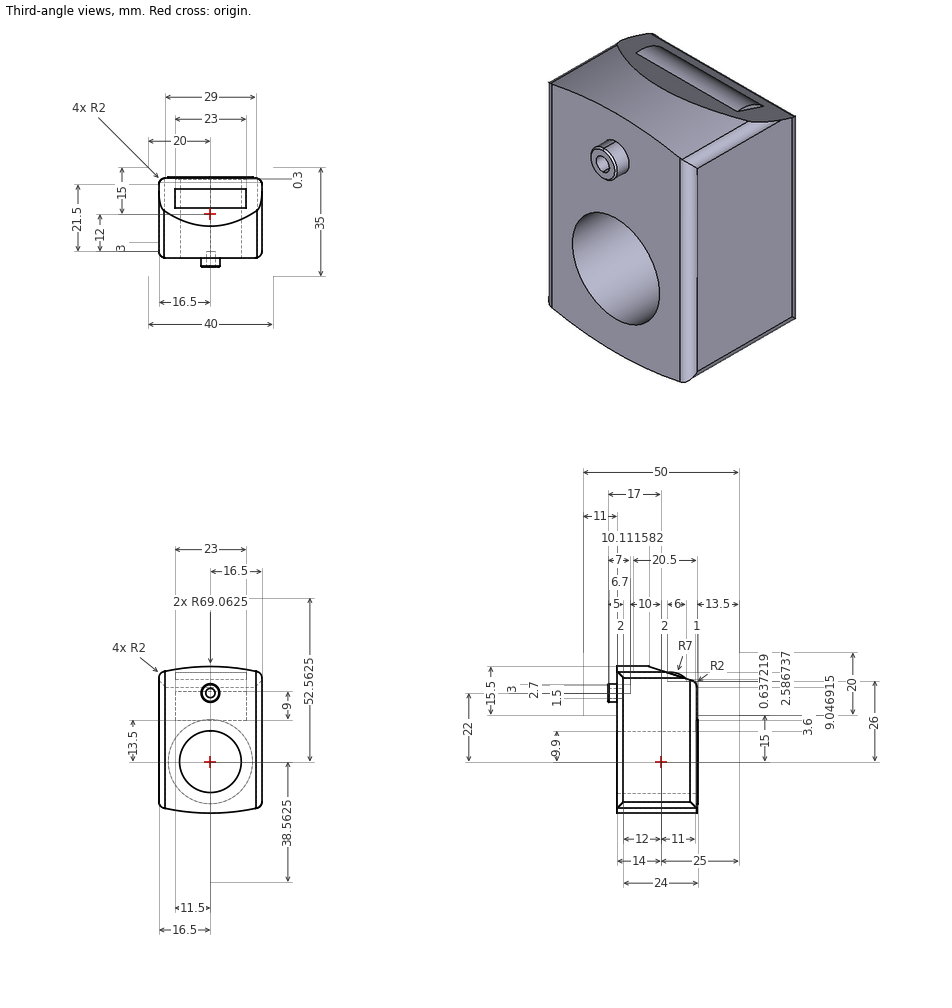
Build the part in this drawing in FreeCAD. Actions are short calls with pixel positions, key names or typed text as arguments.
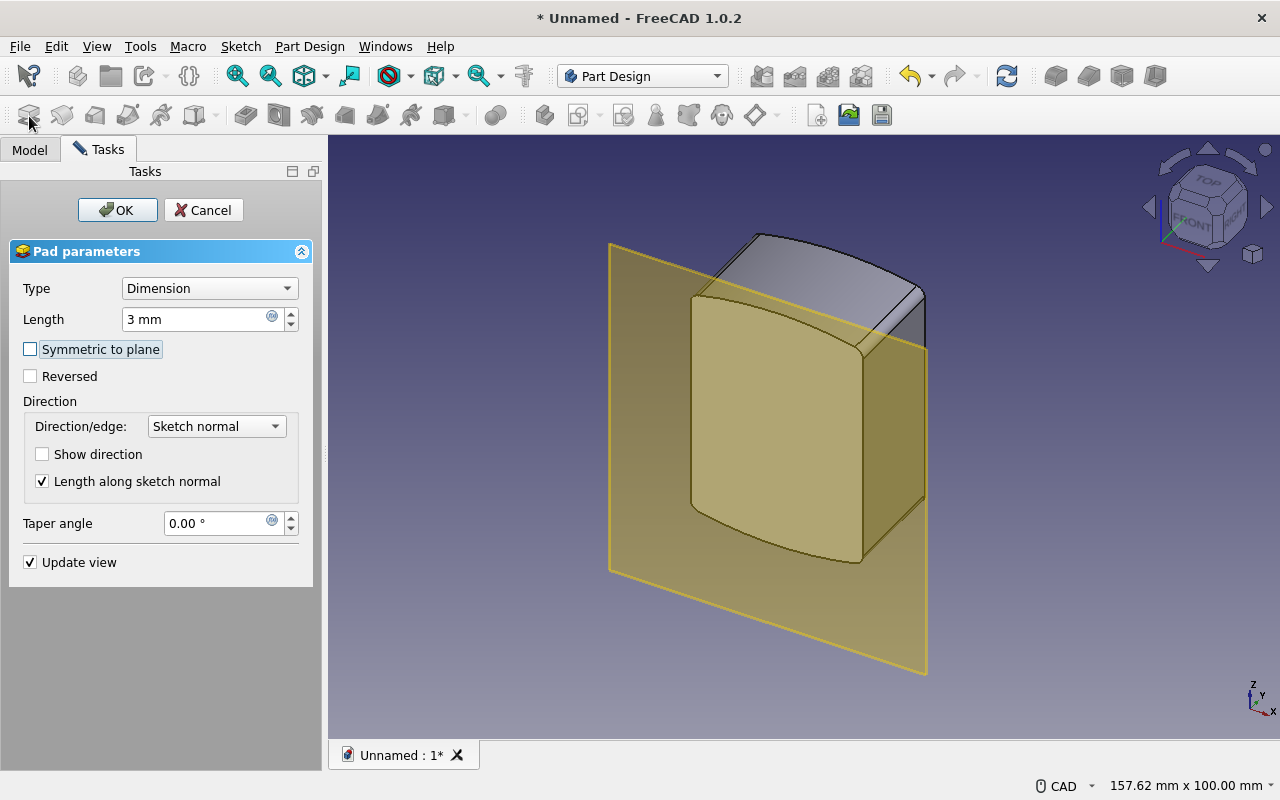
click(31, 376)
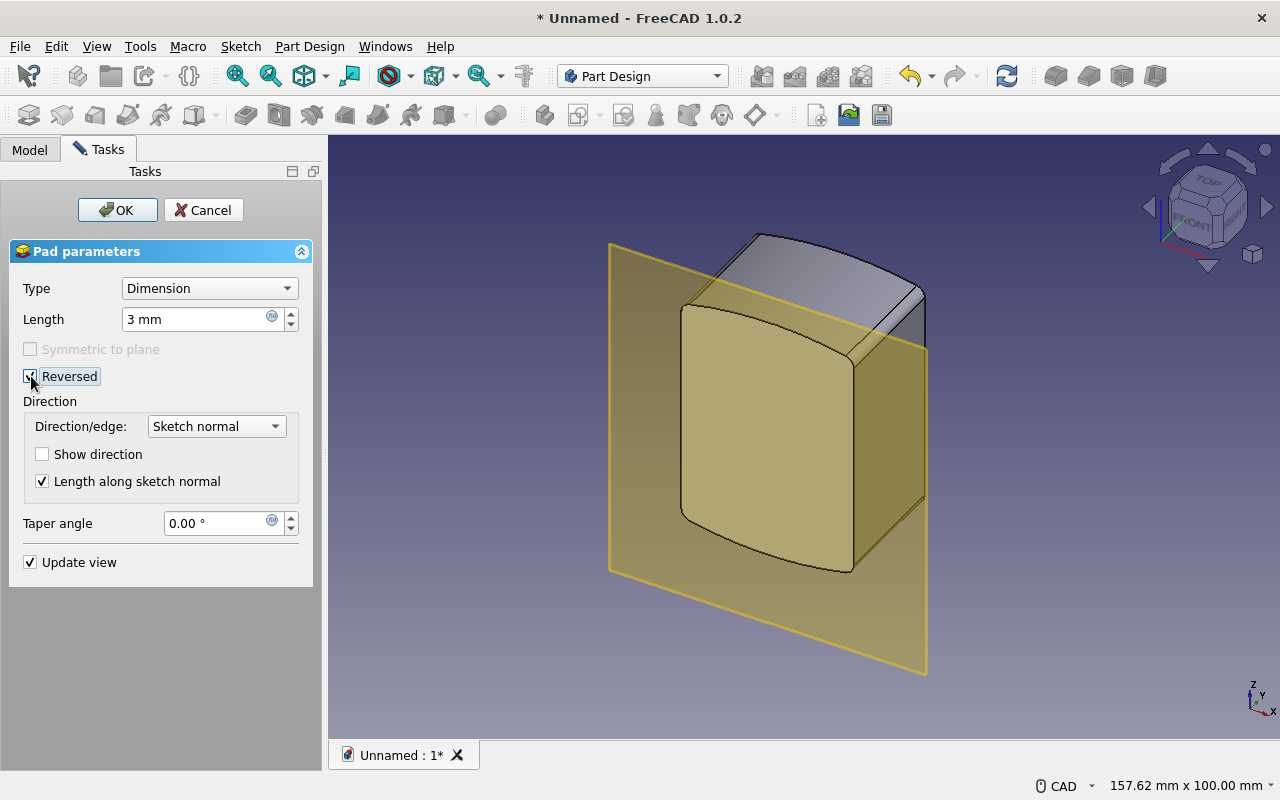
click(118, 210)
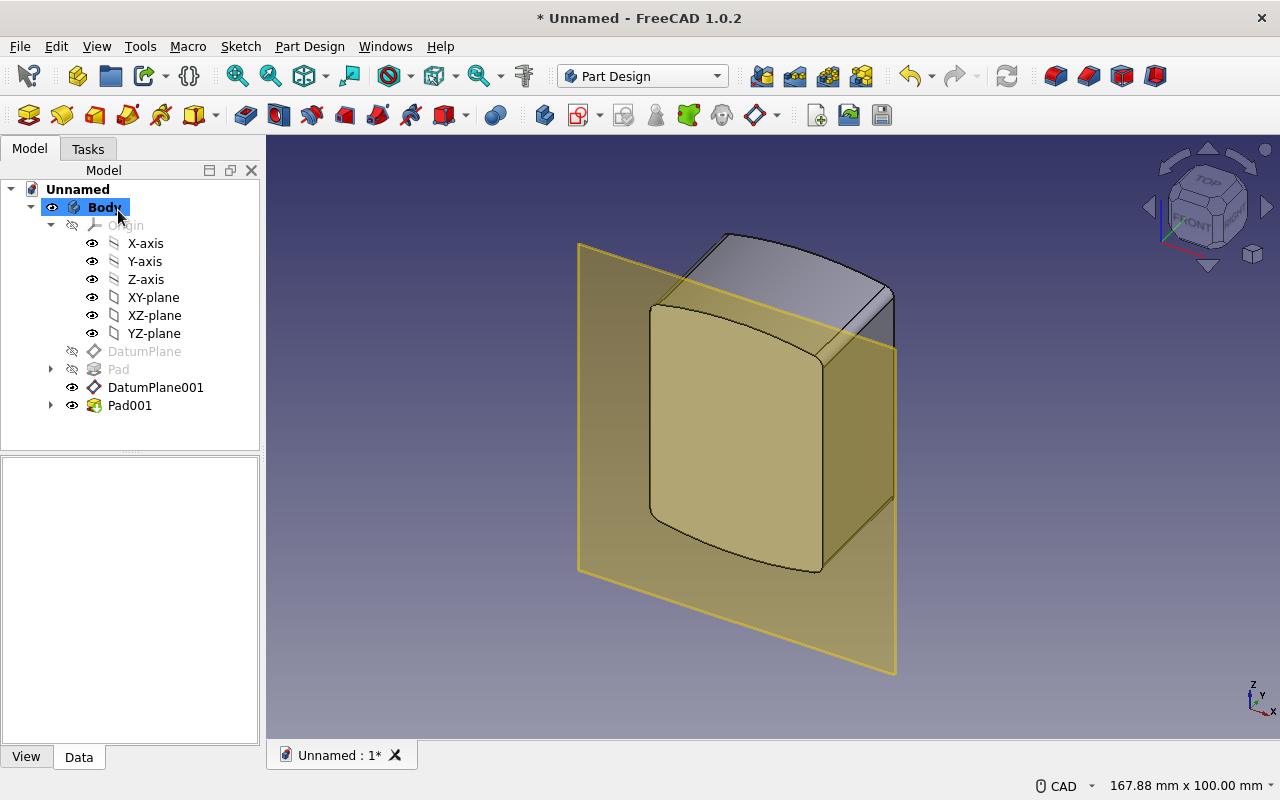
click(117, 387)
key(space)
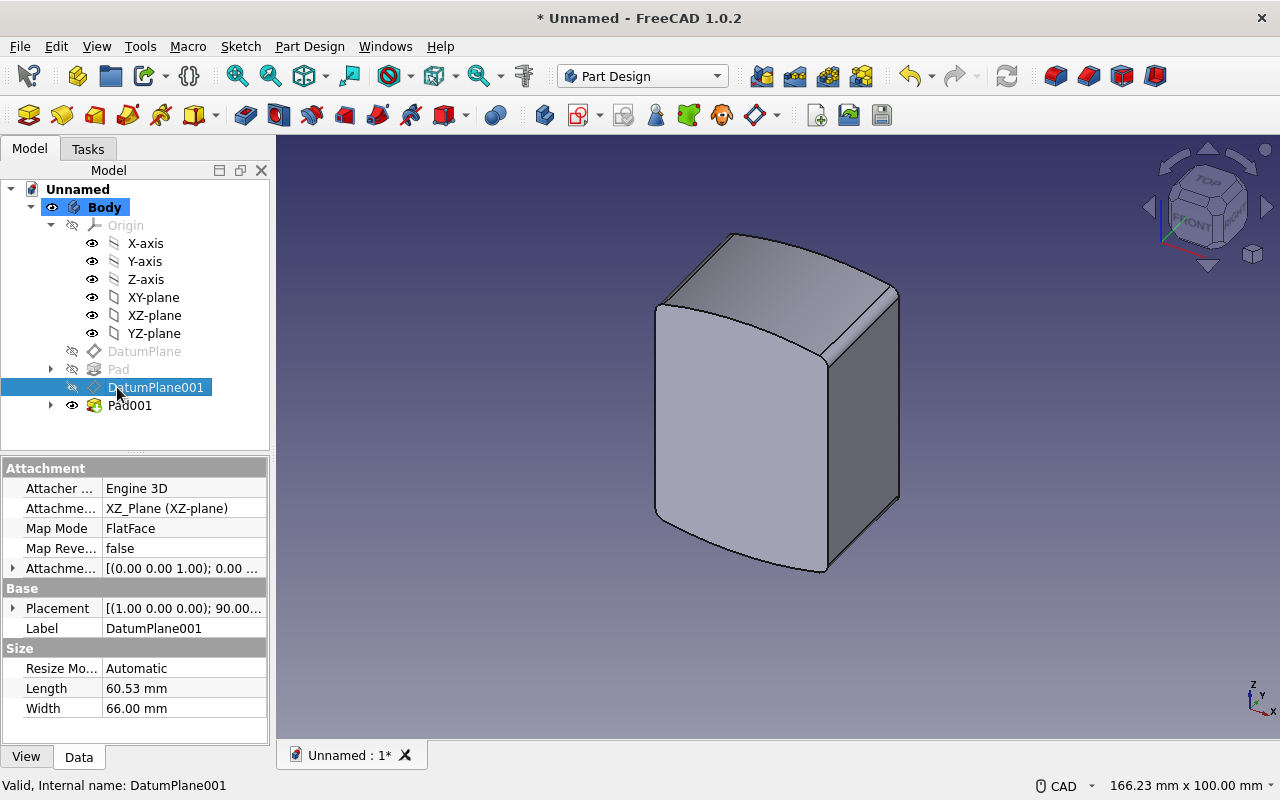
click(137, 315)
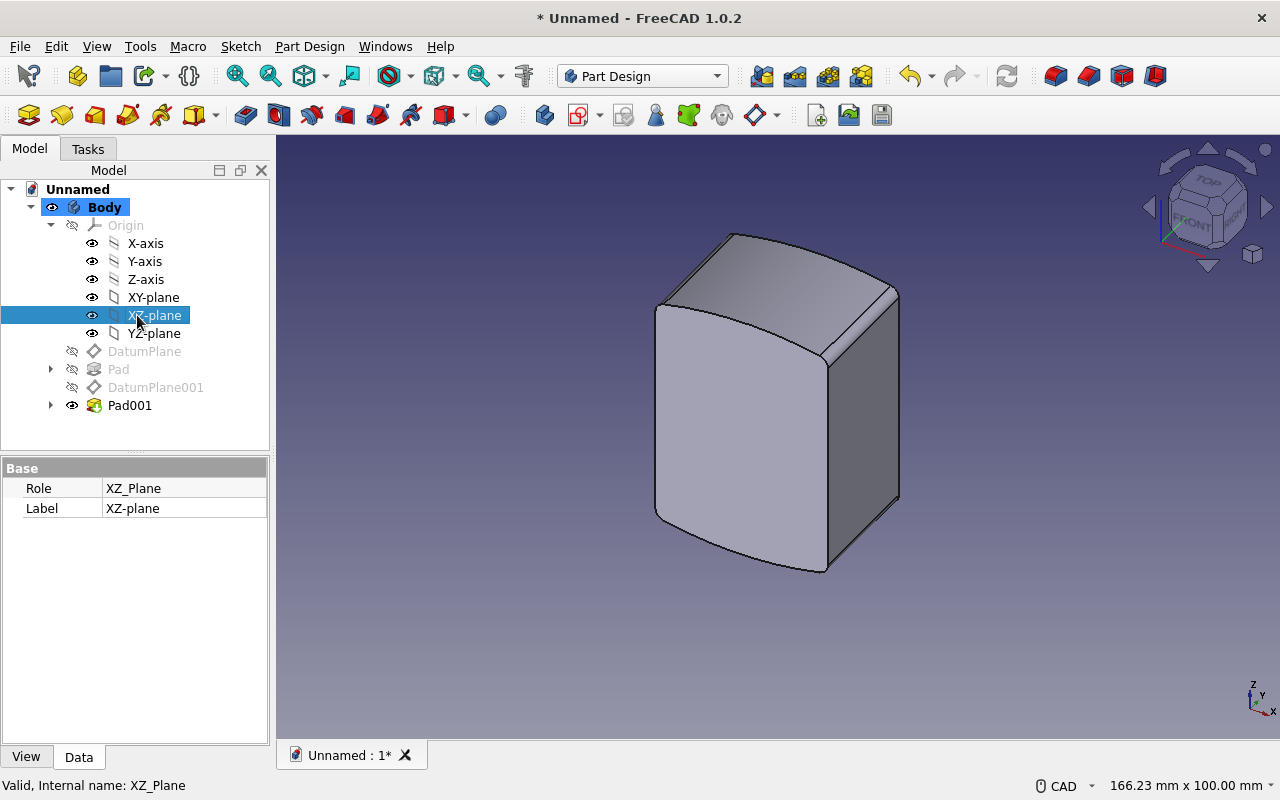
click(754, 116)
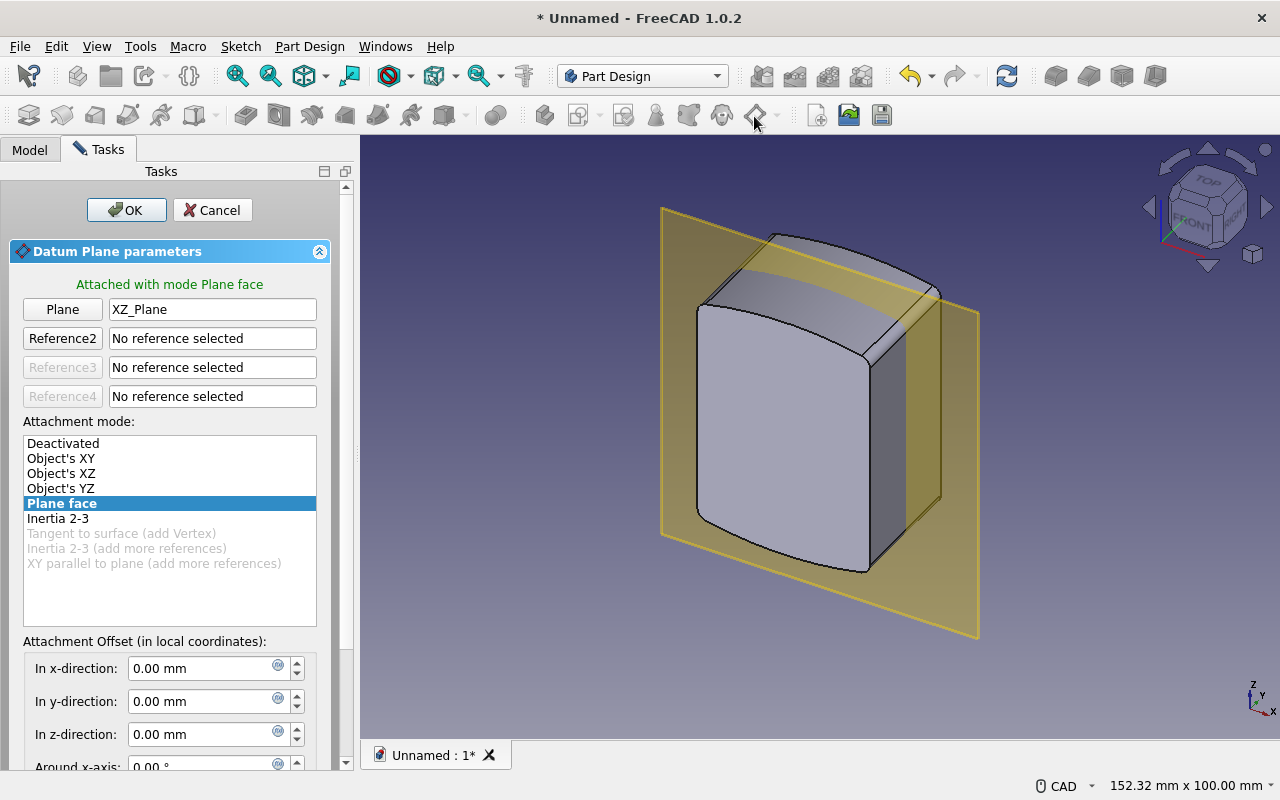
triple_click(210, 734)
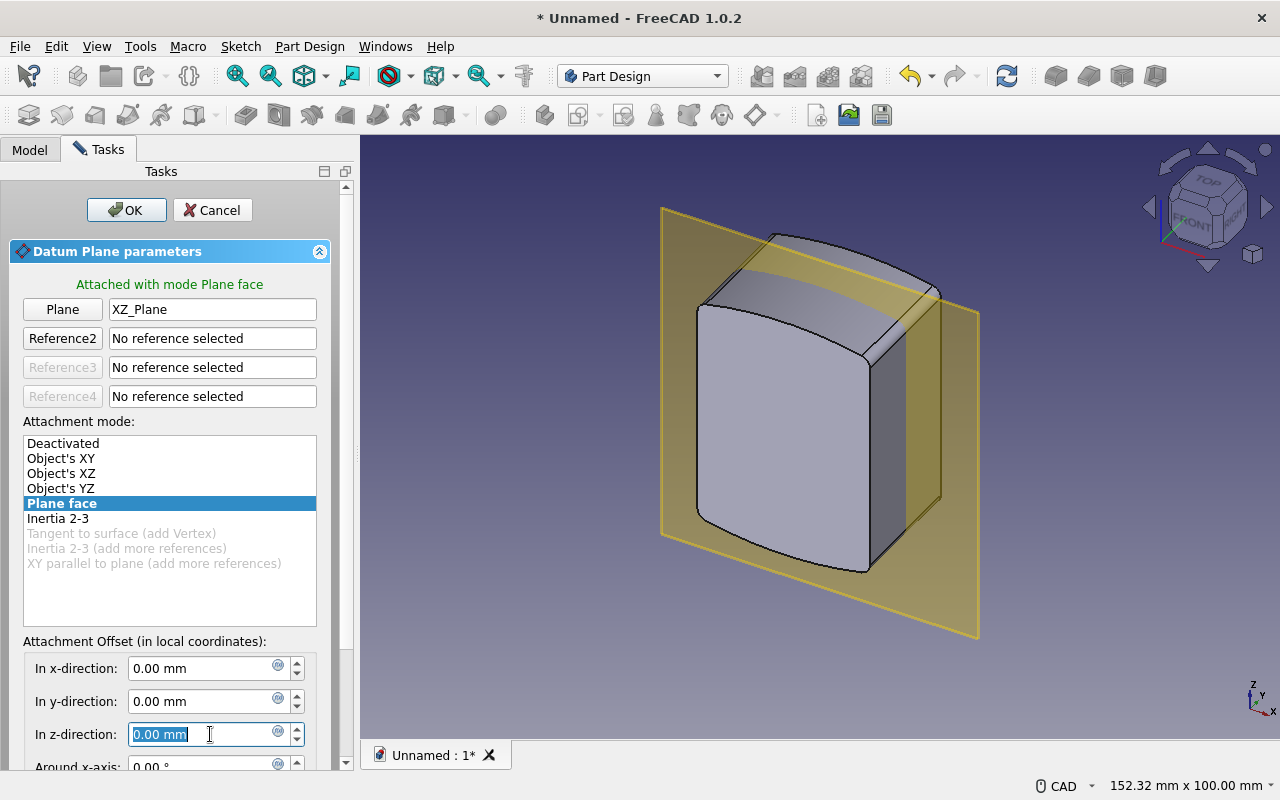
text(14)
key(Tab)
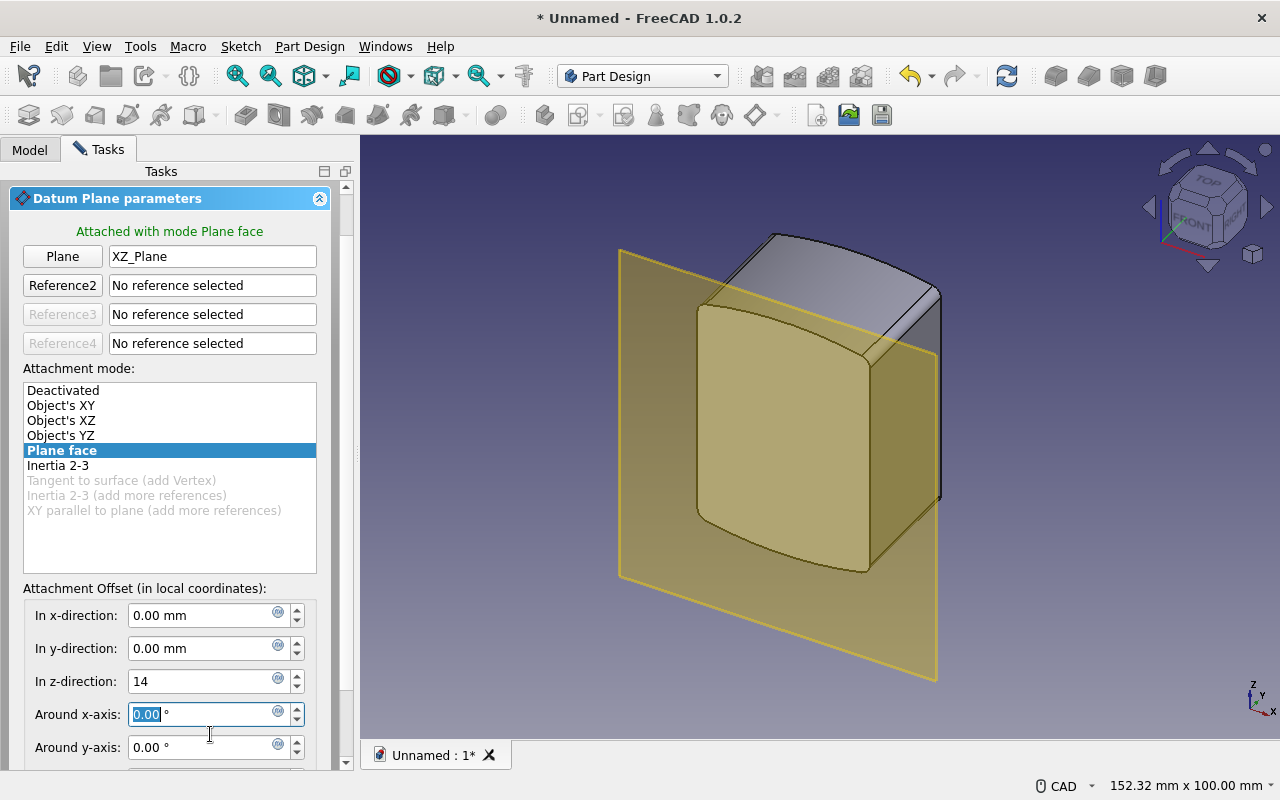
scroll(346, 476, up, 2)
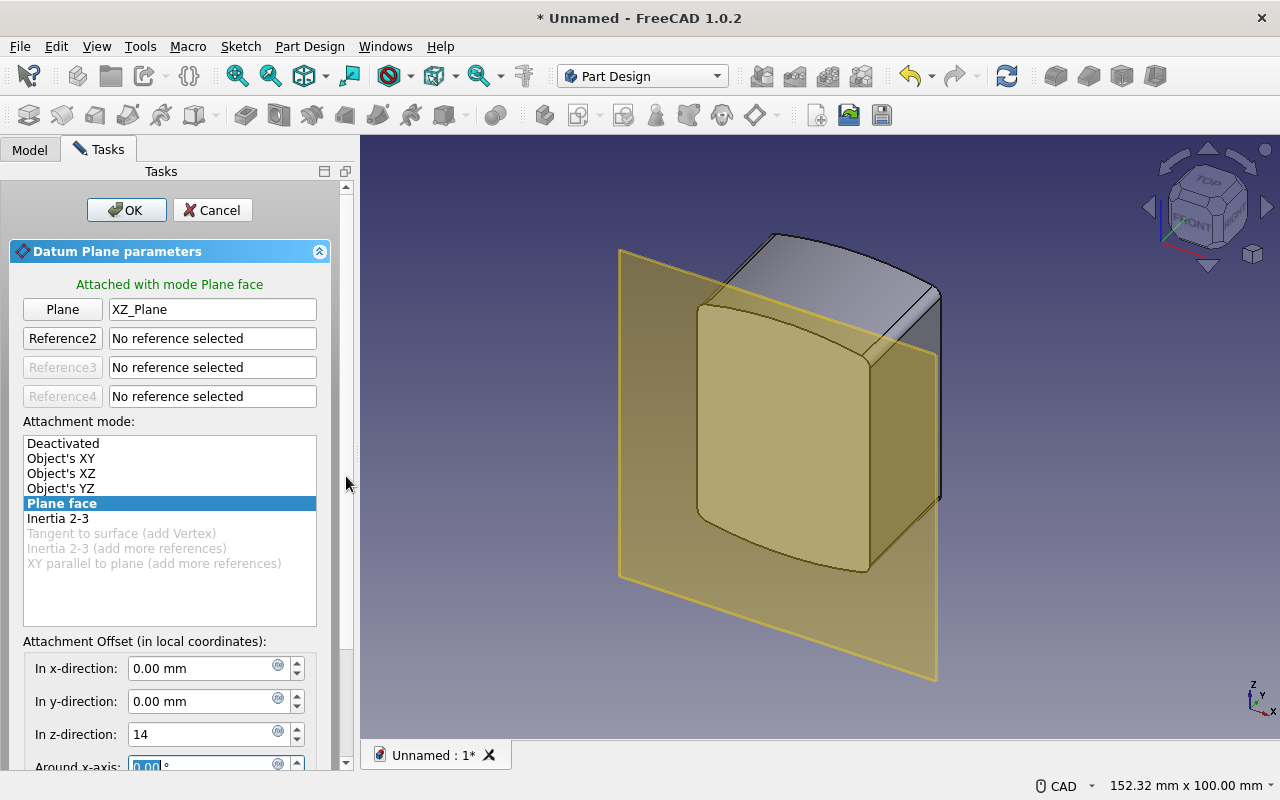
click(127, 210)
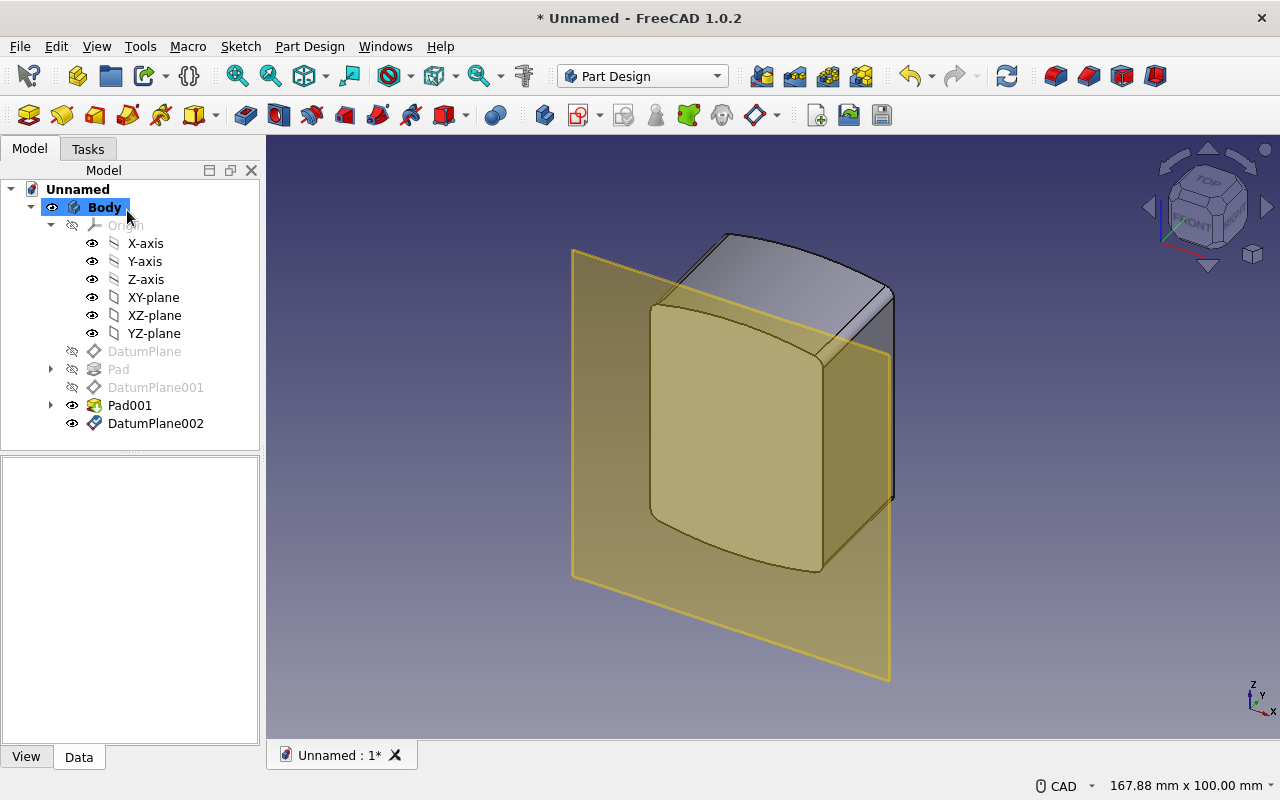
click(117, 423)